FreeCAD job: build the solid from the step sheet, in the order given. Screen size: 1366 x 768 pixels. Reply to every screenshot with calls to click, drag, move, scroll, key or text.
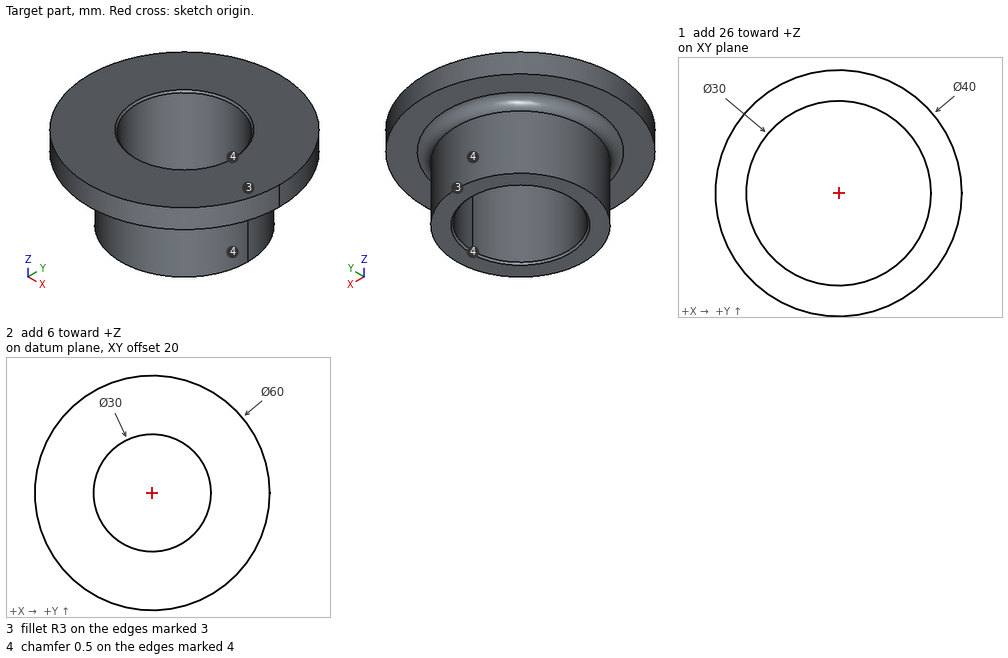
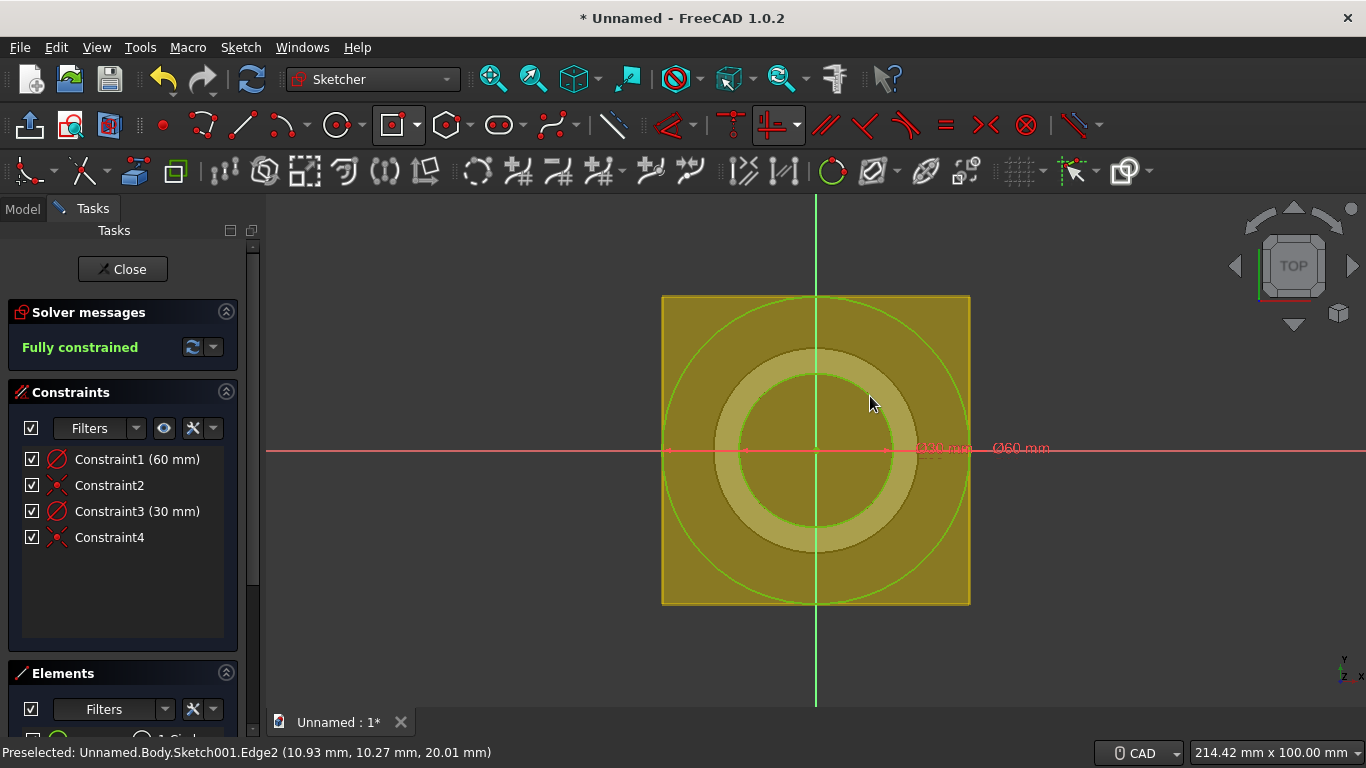
click(123, 269)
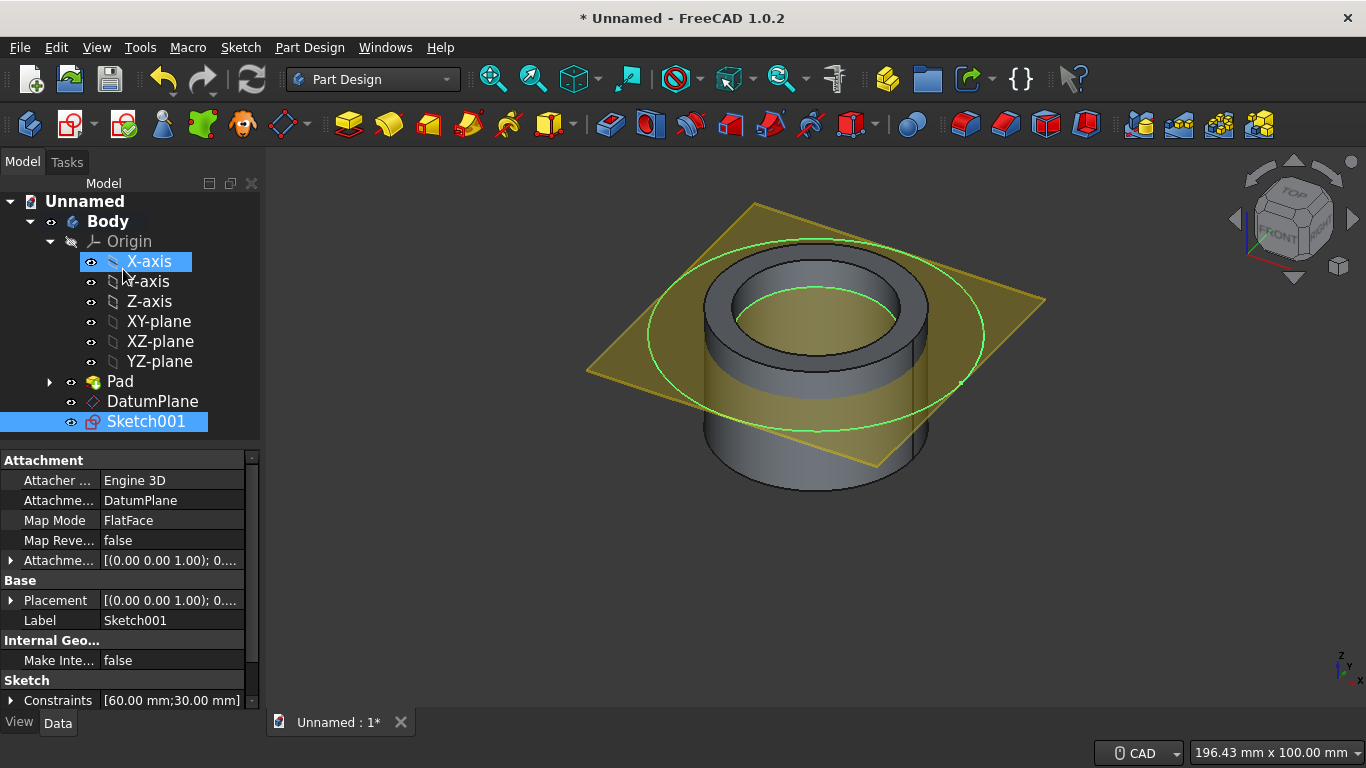
click(350, 124)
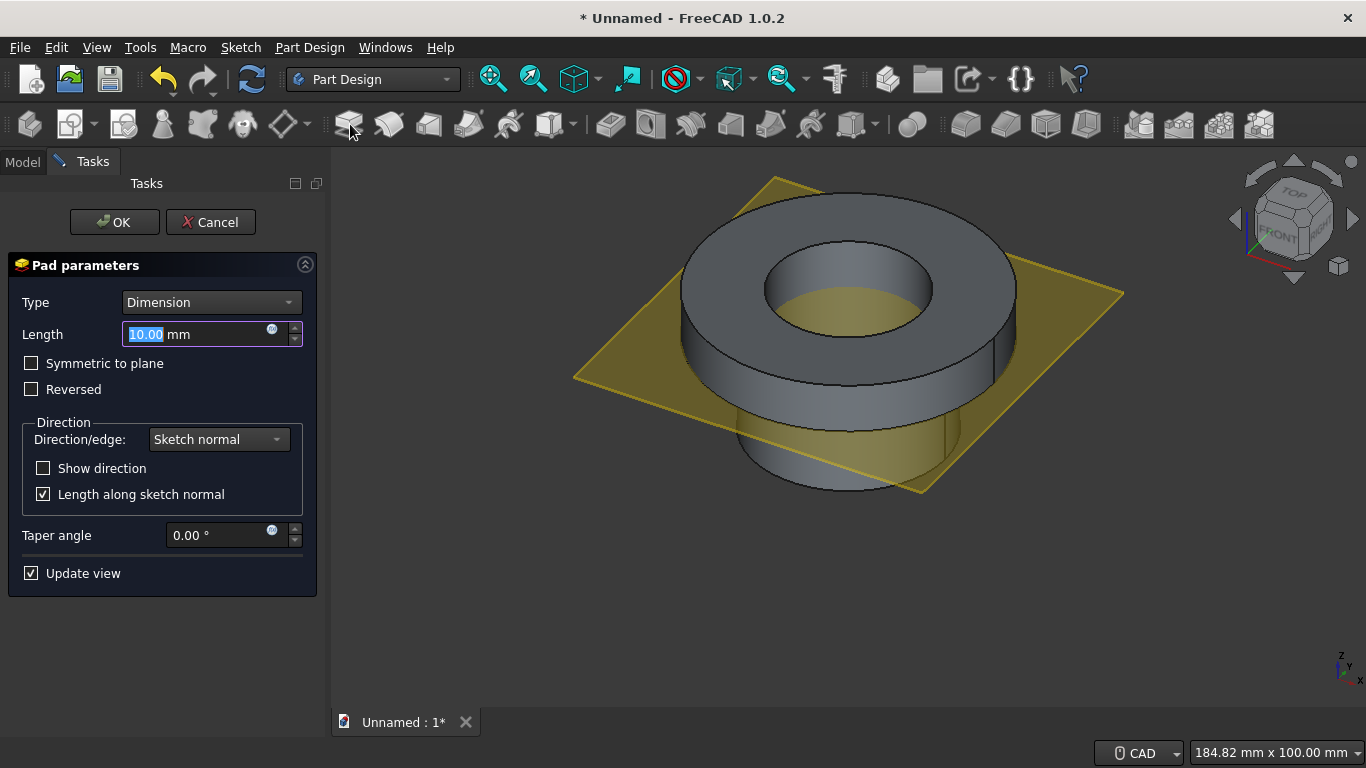
text(6)
key(Tab)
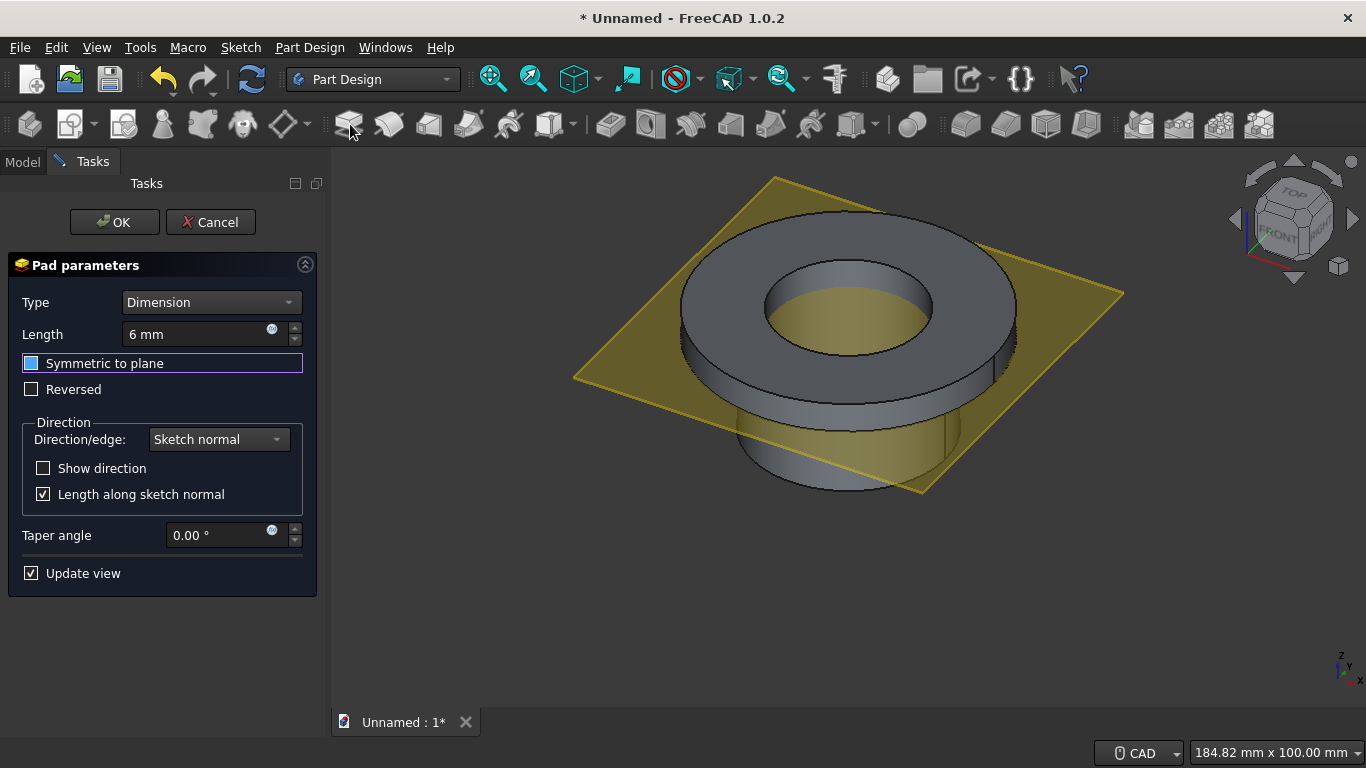
click(115, 222)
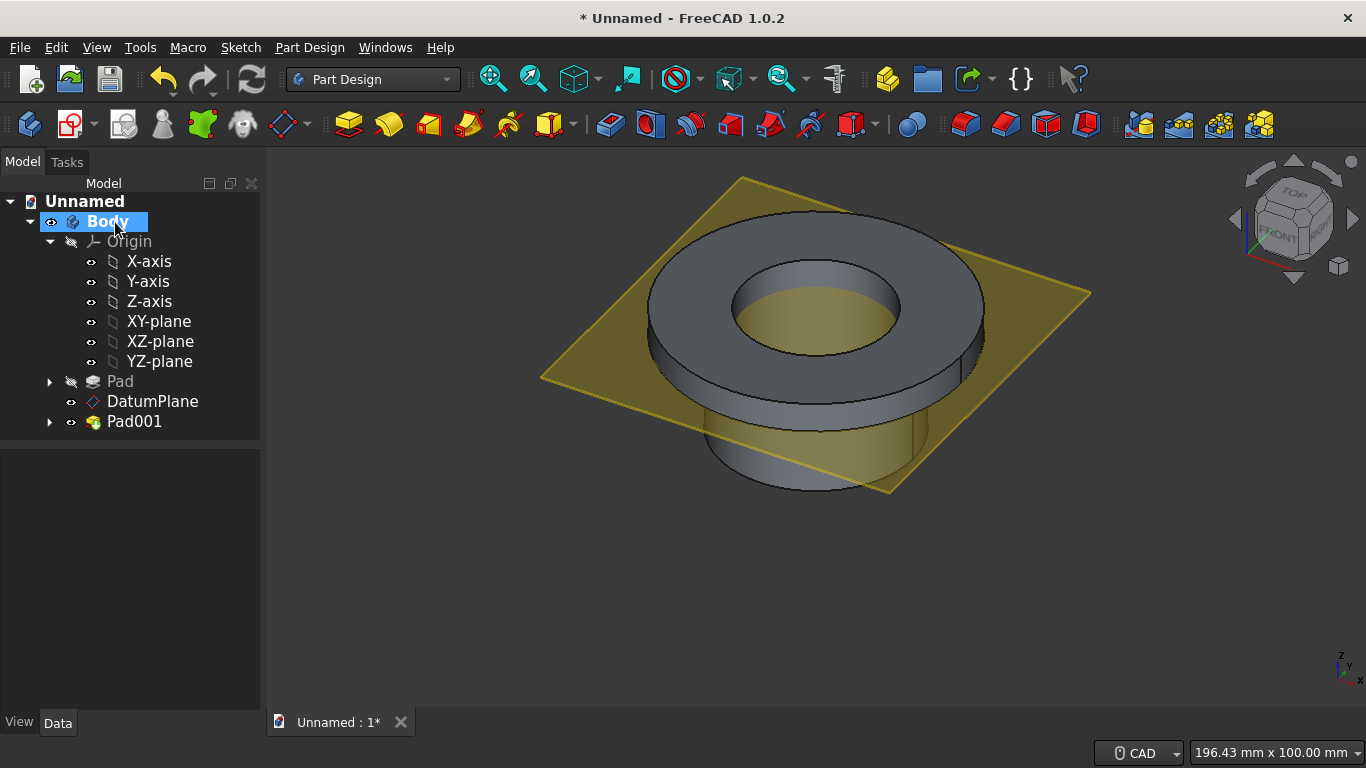
click(116, 402)
key(space)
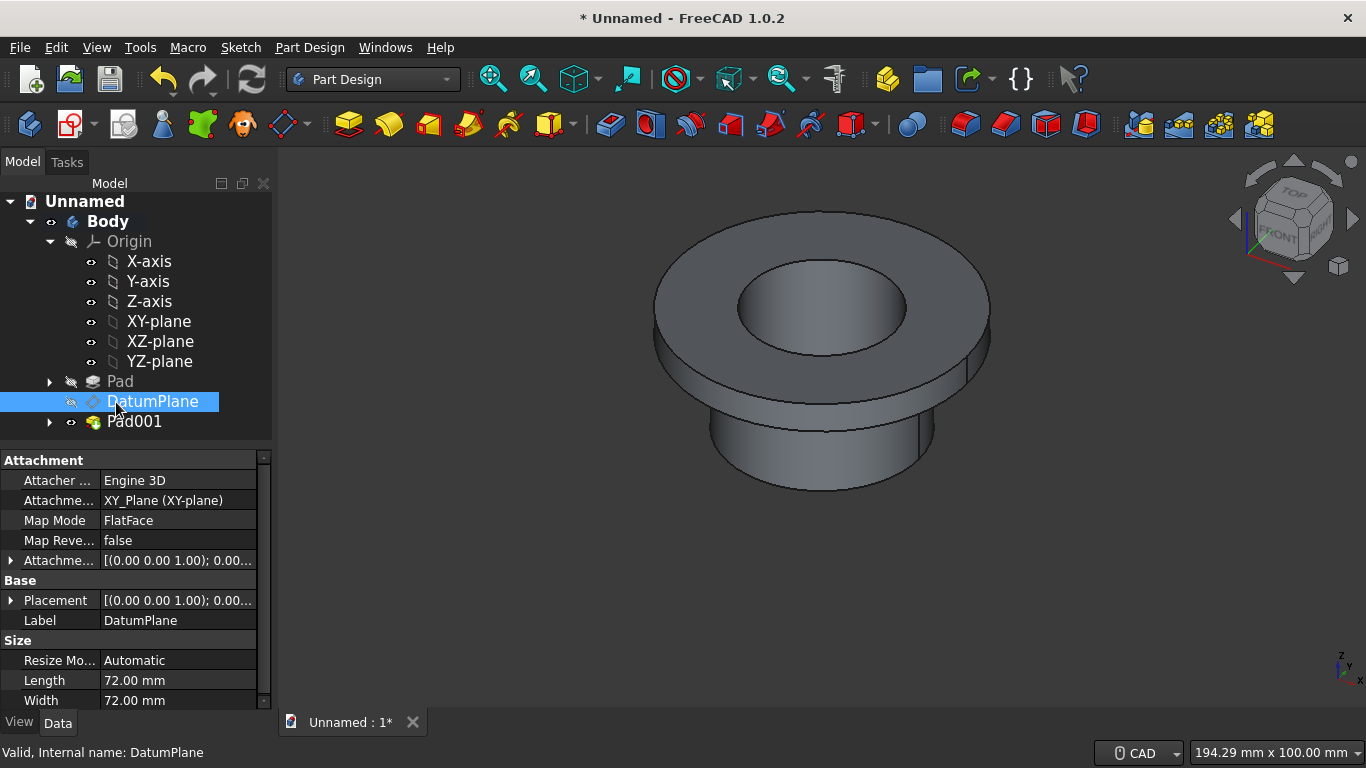
key(0)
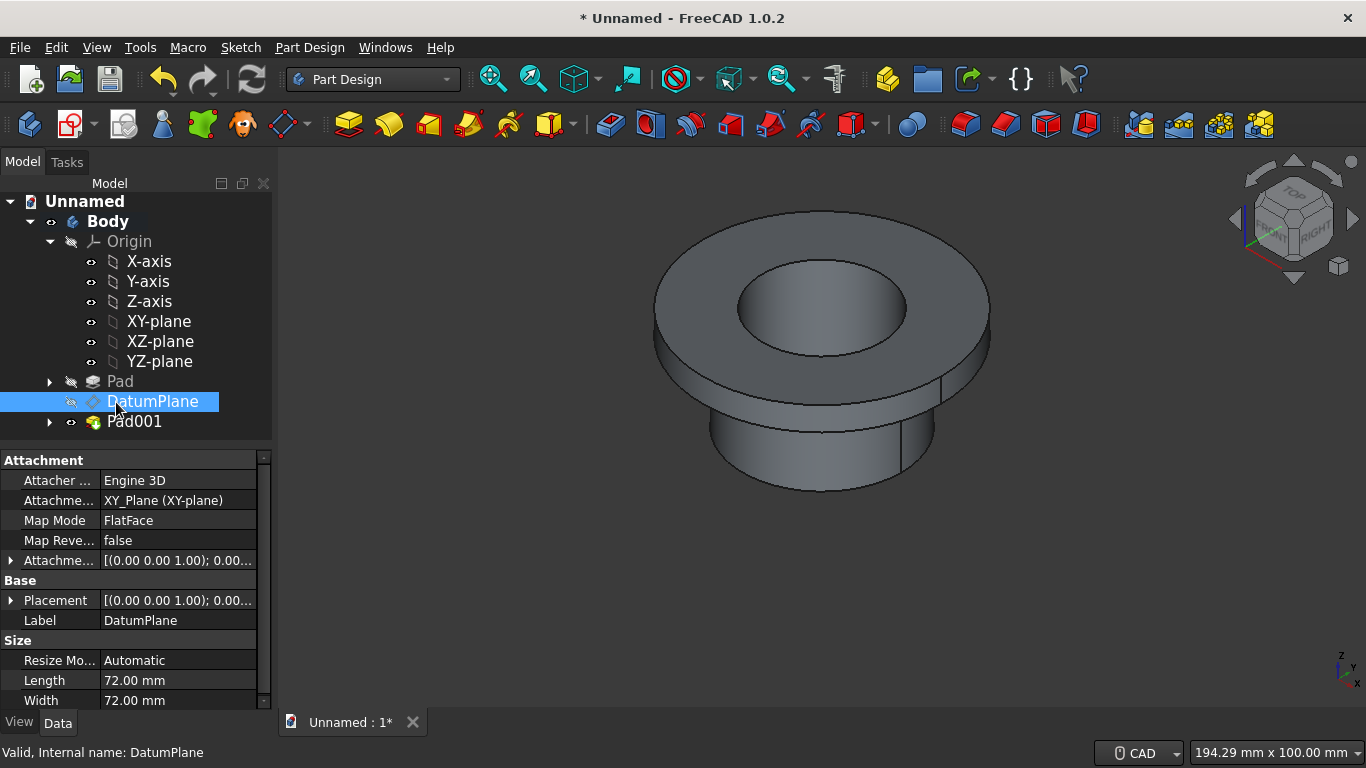
key(2)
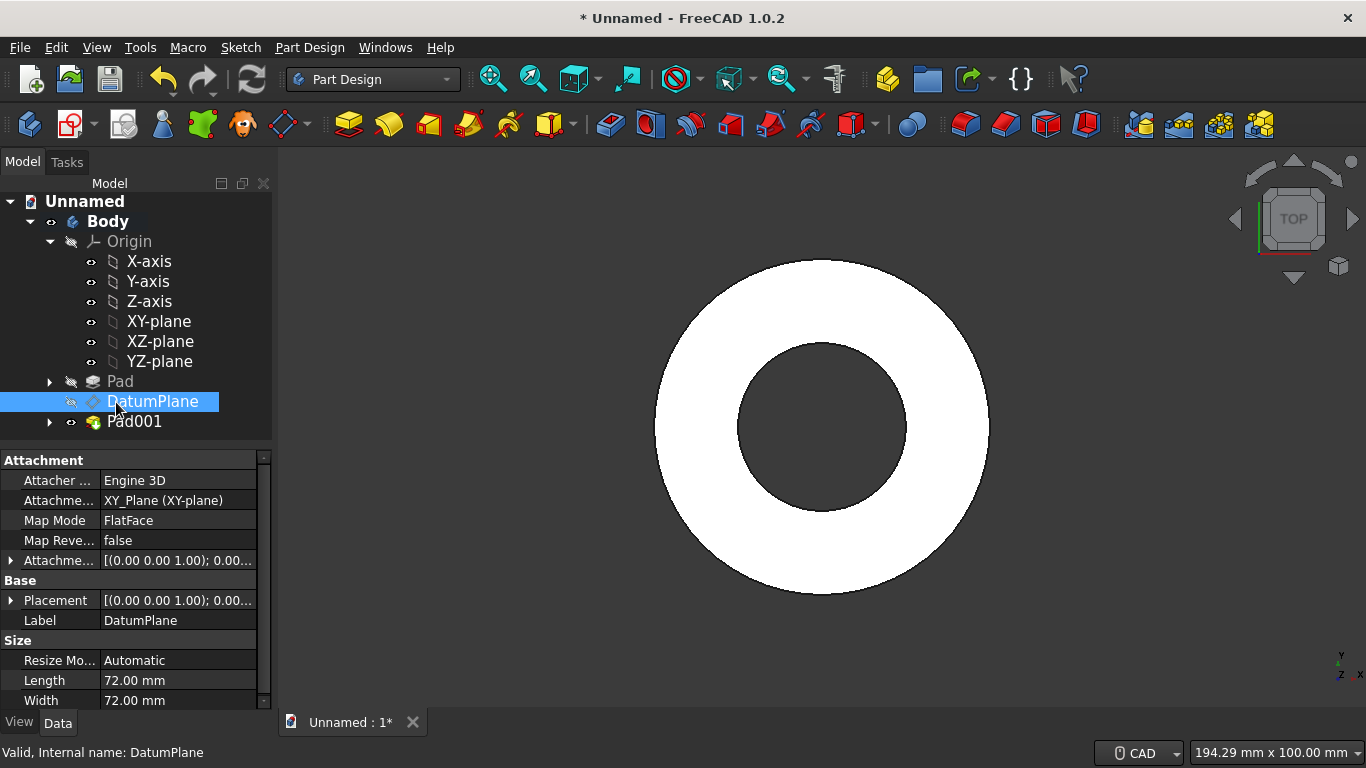
key(1)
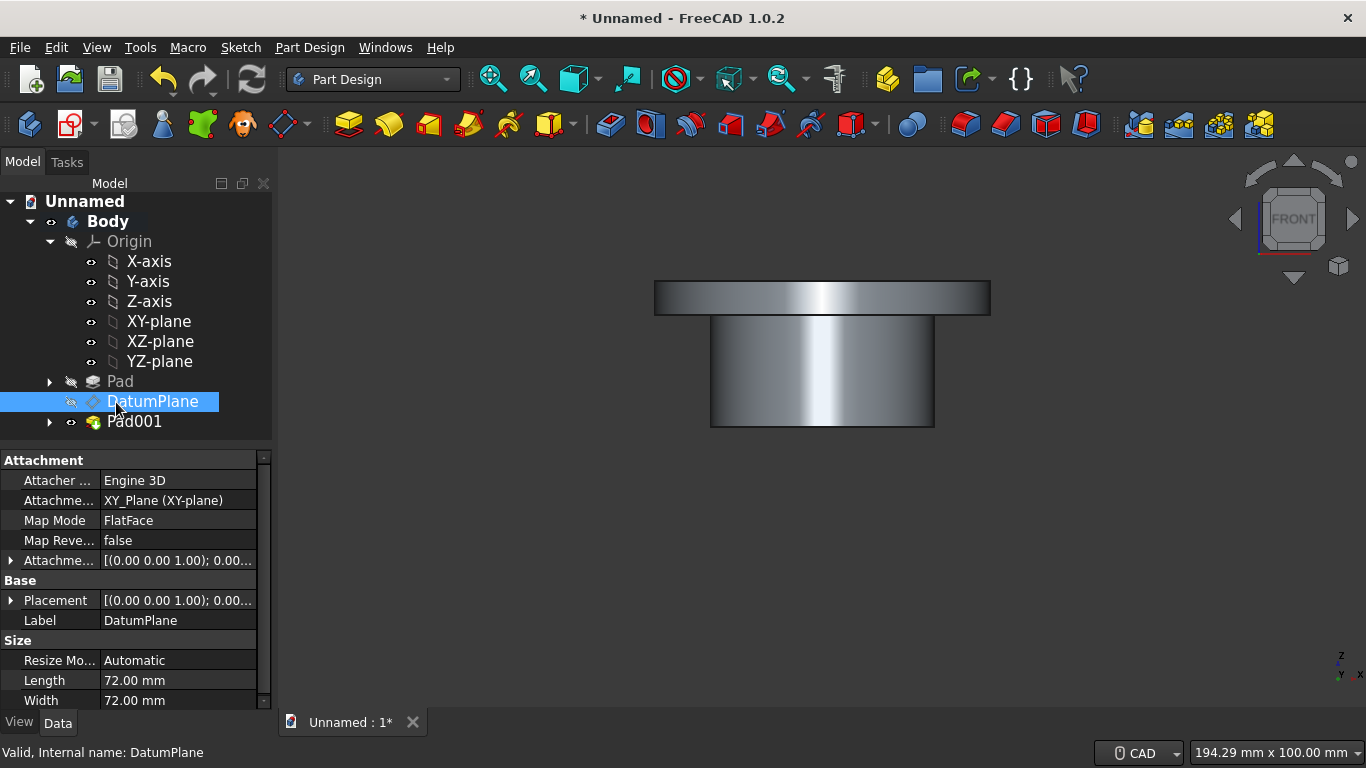
click(494, 80)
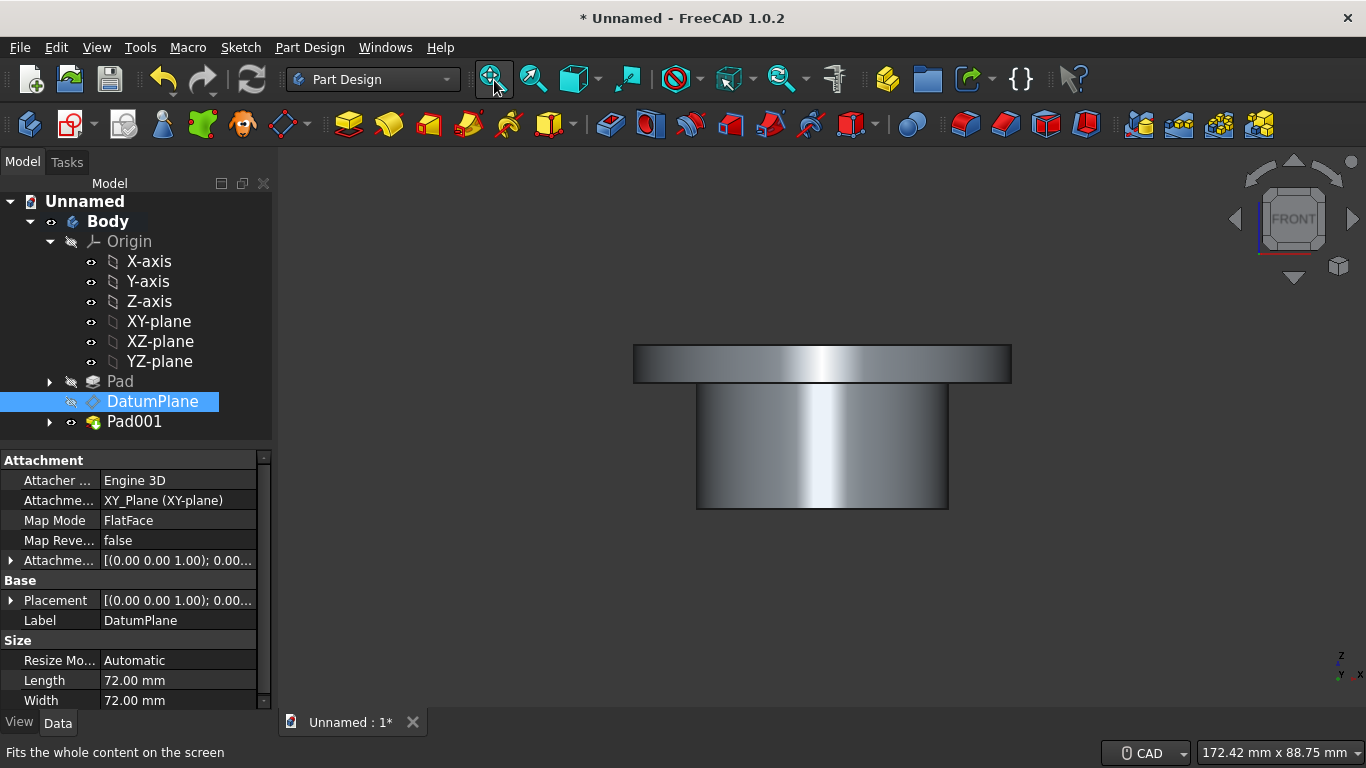
key(3)